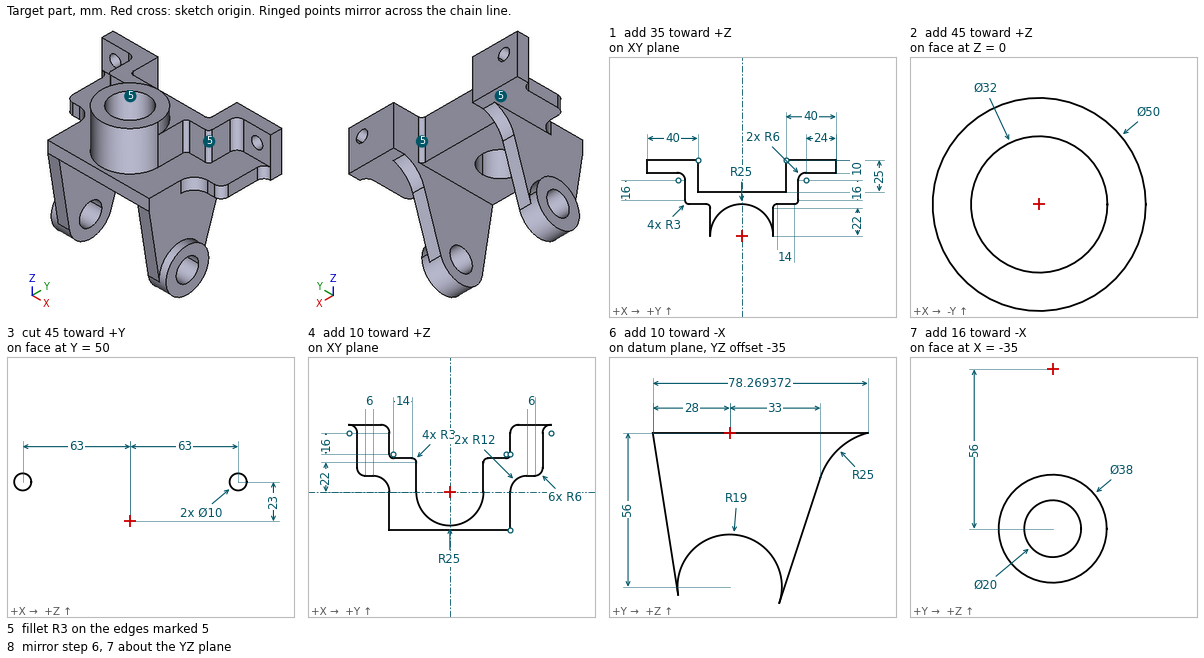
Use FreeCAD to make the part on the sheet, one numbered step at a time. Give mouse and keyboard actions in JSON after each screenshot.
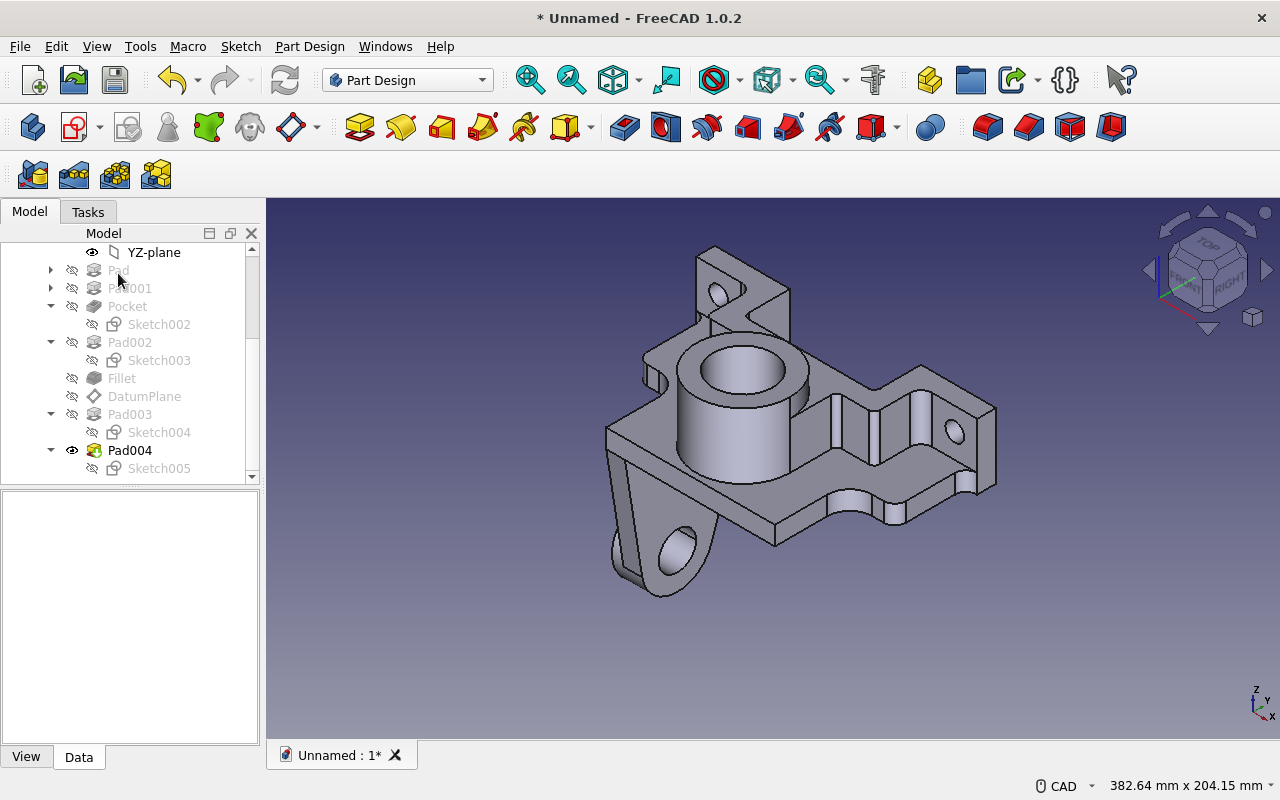
{"action": "left_click", "coordinate": [531, 80]}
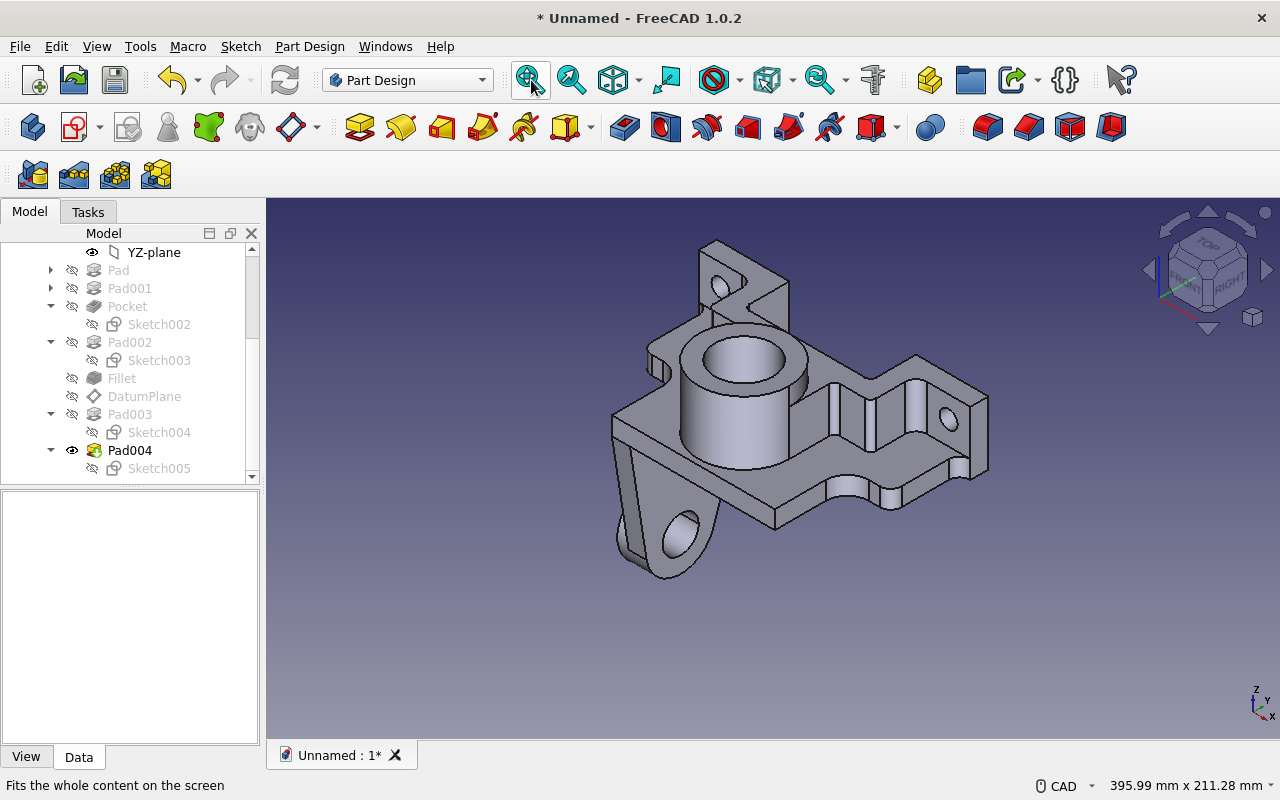
{"action": "left_click", "coordinate": [117, 414]}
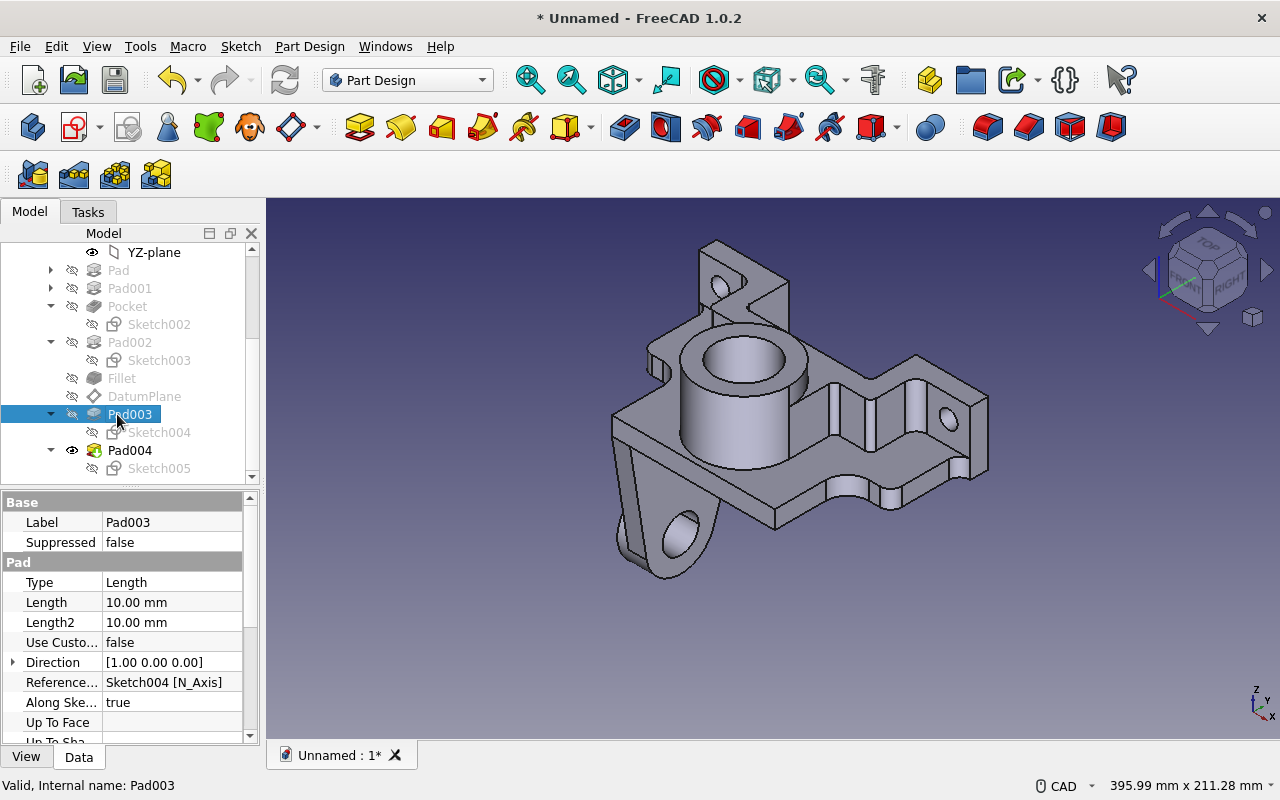
{"action": "left_click", "coordinate": [117, 450], "text": "ctrl"}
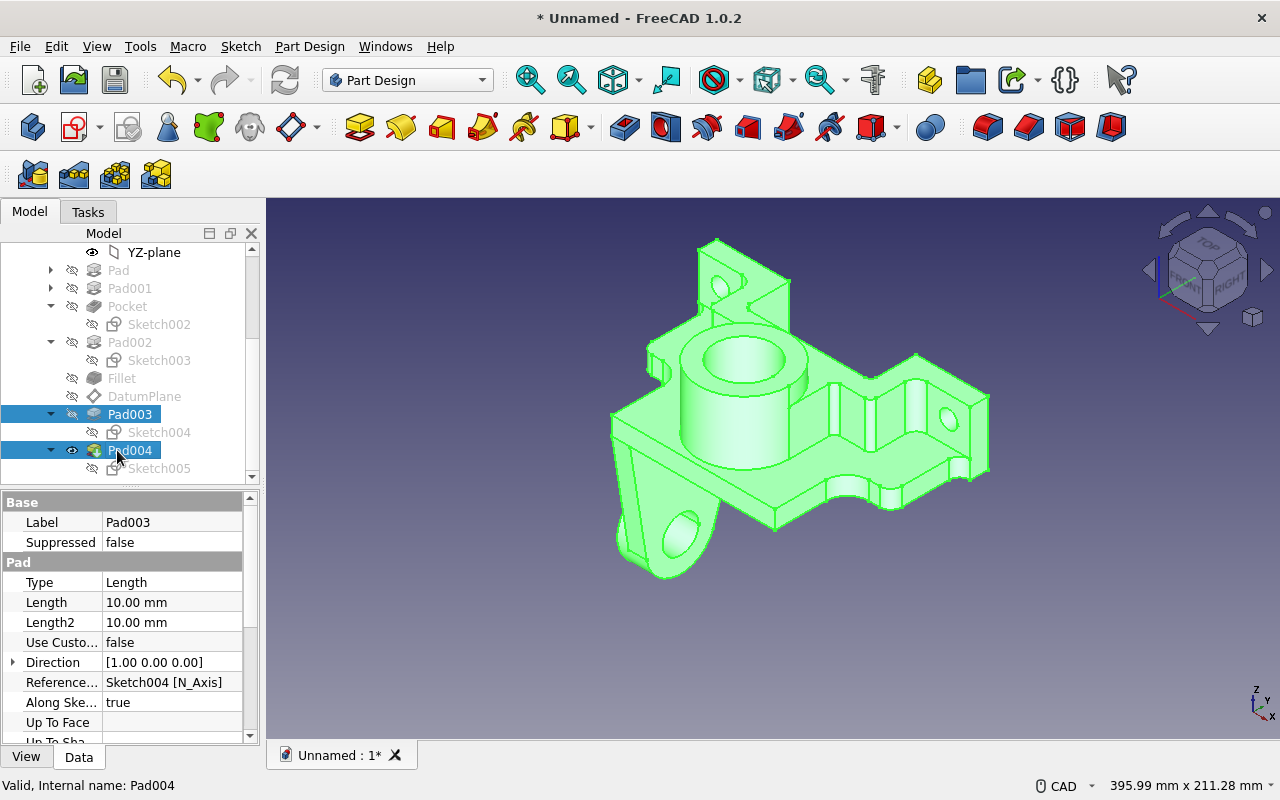
{"action": "left_click", "coordinate": [33, 174]}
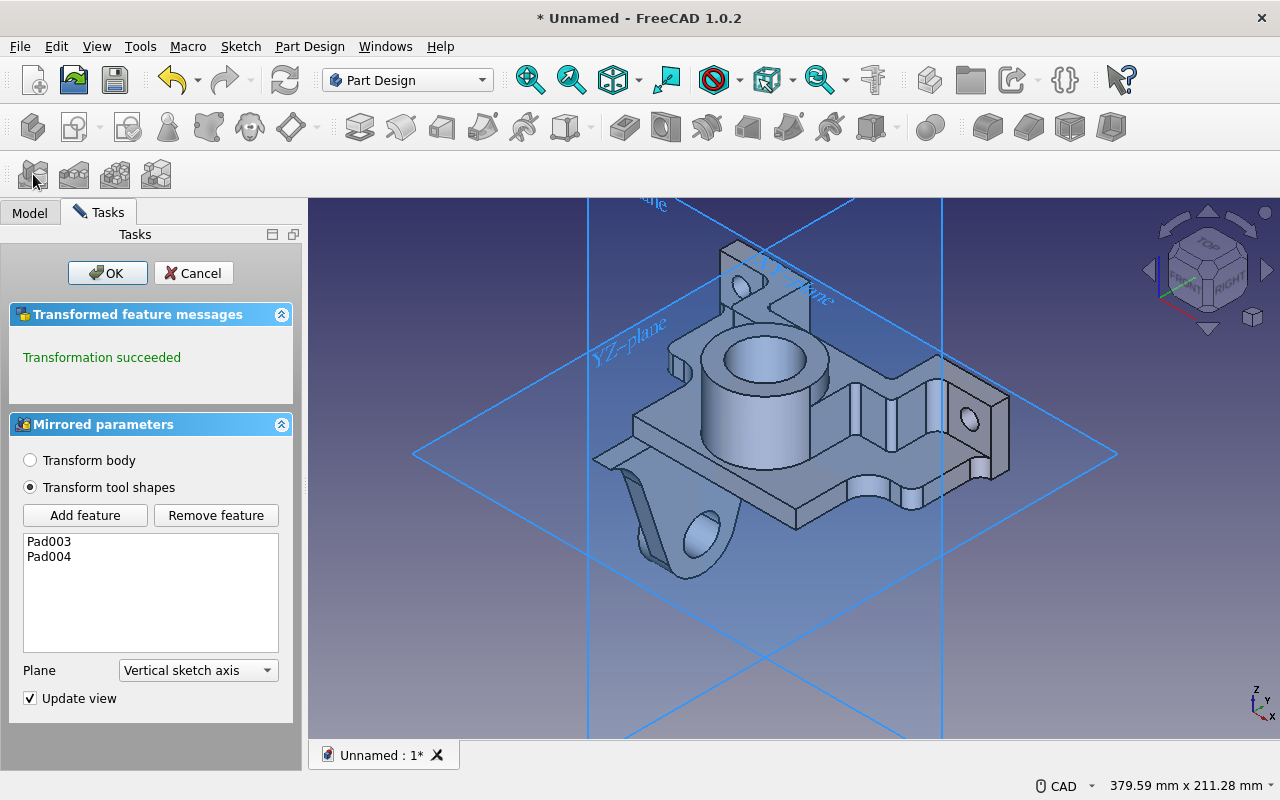
{"action": "left_click", "coordinate": [199, 670]}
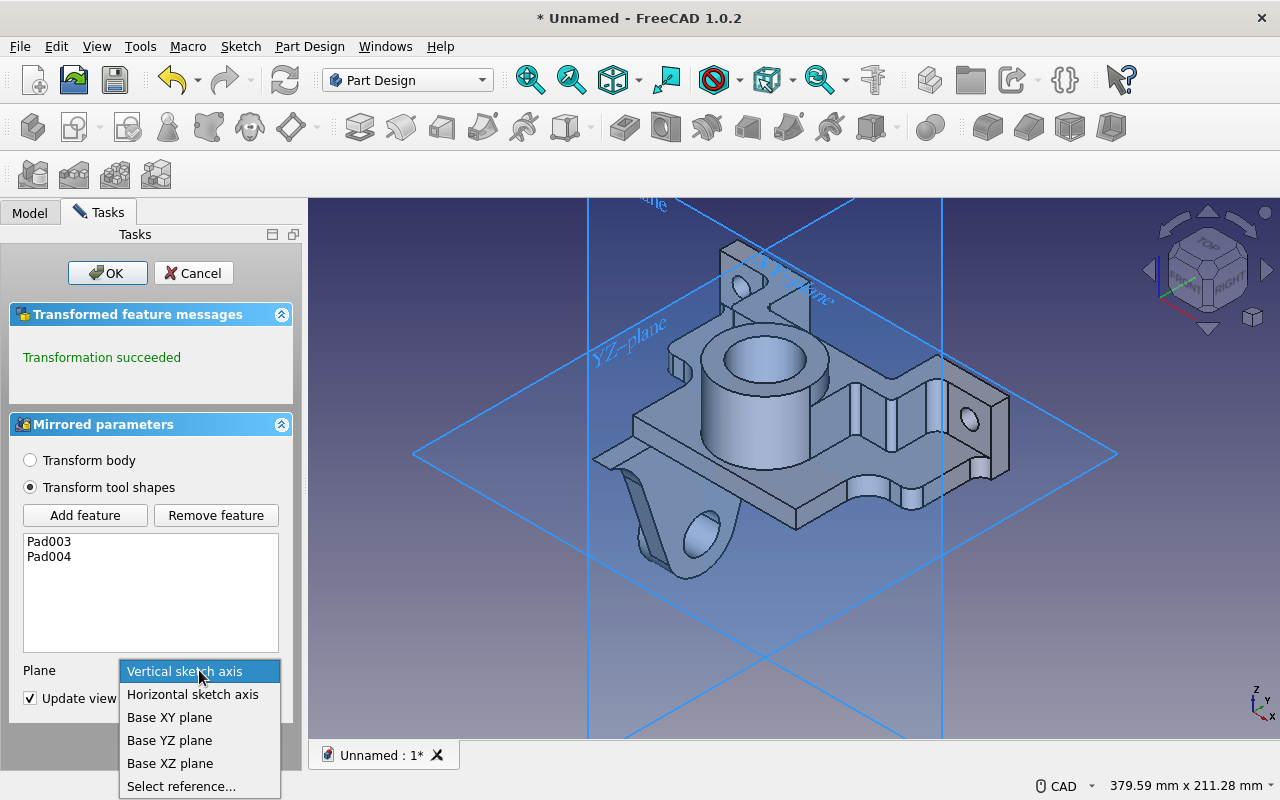
{"action": "left_click", "coordinate": [198, 740]}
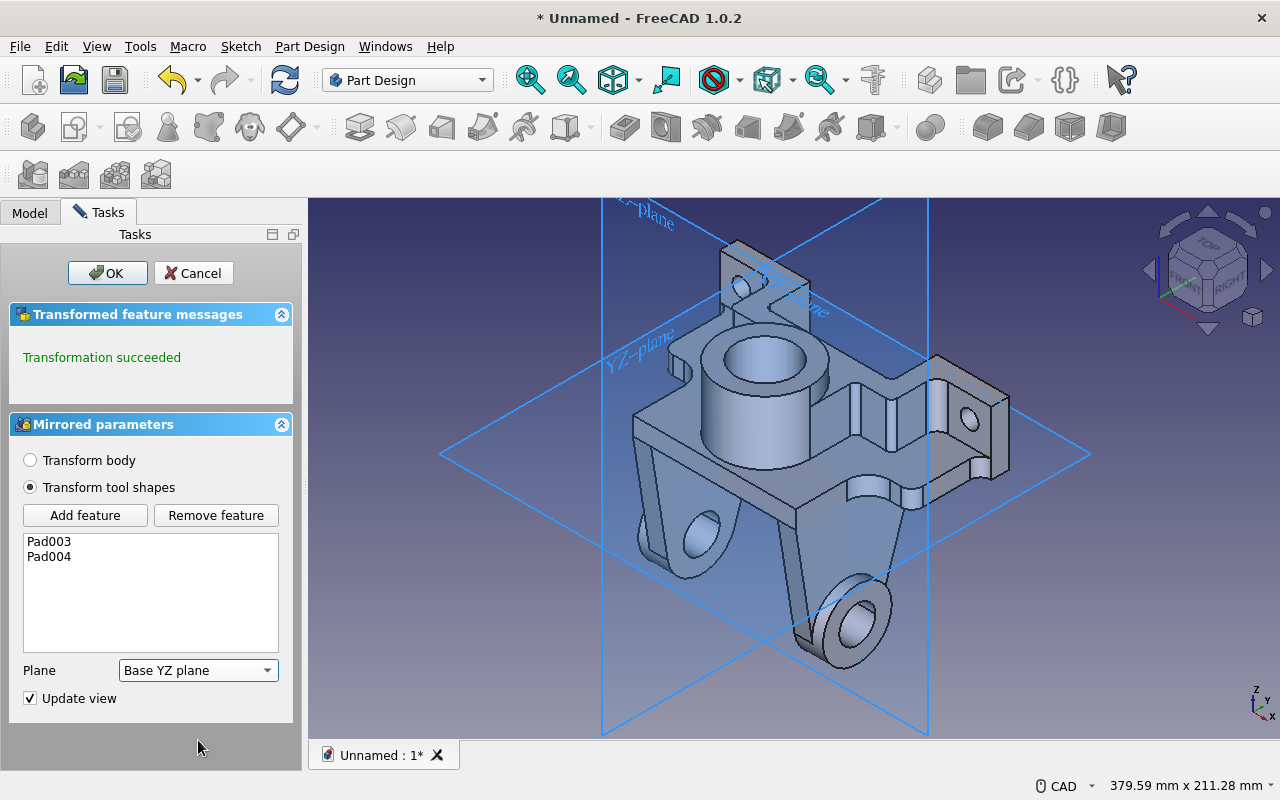
{"action": "left_click", "coordinate": [108, 273]}